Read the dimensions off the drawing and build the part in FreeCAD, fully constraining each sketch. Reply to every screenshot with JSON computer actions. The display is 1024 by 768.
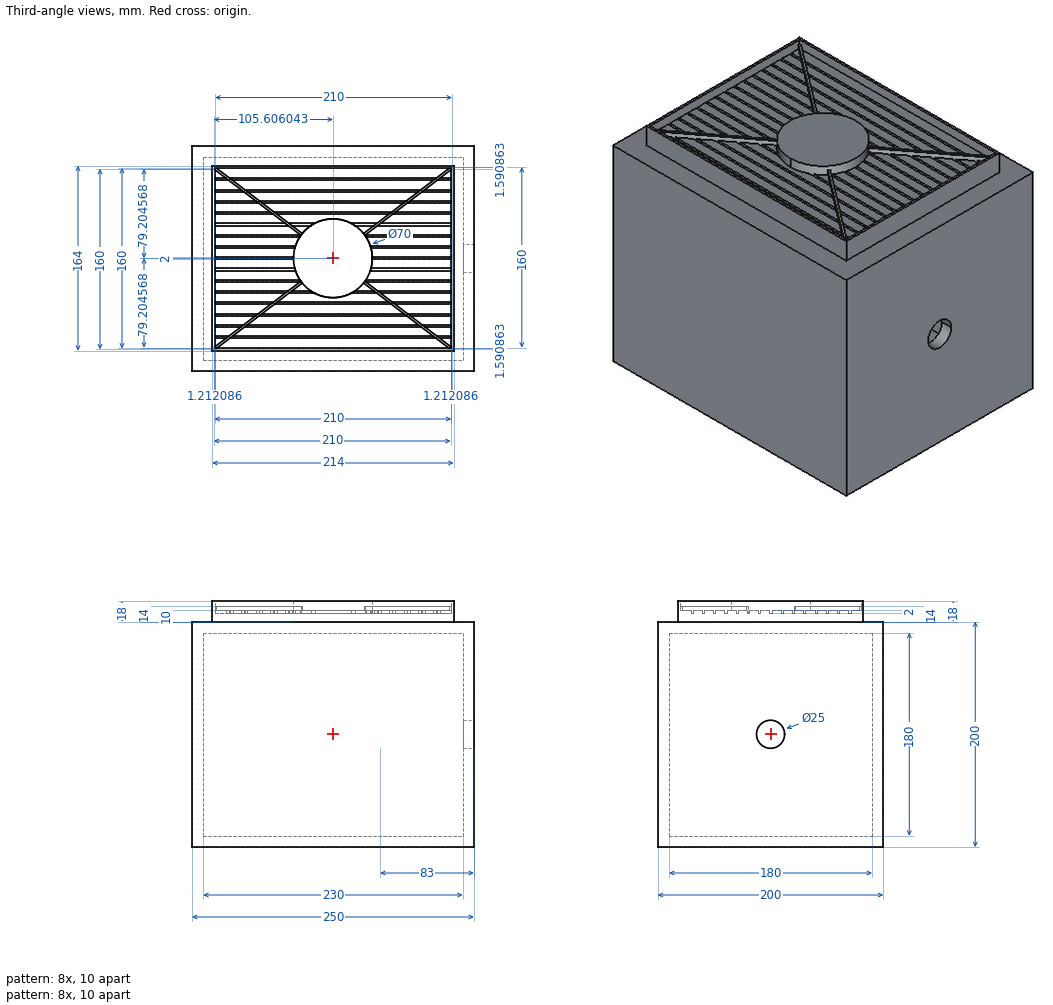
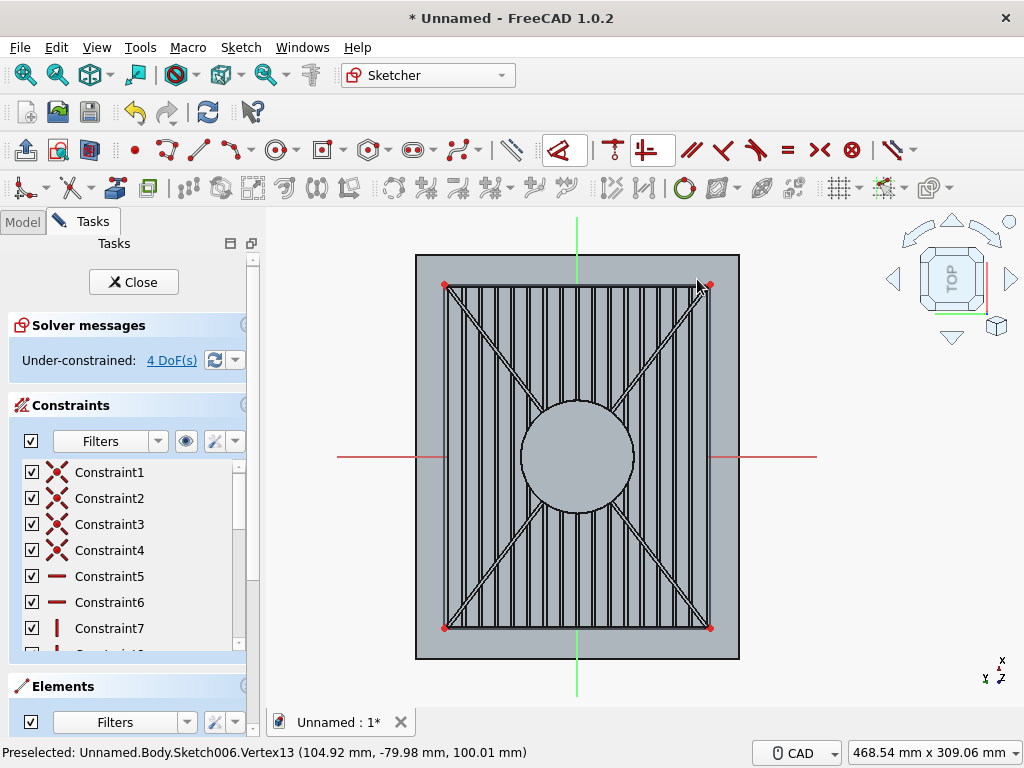
{"action": "scroll", "coordinate": [524, 629], "scroll_direction": "up", "scroll_amount": 10}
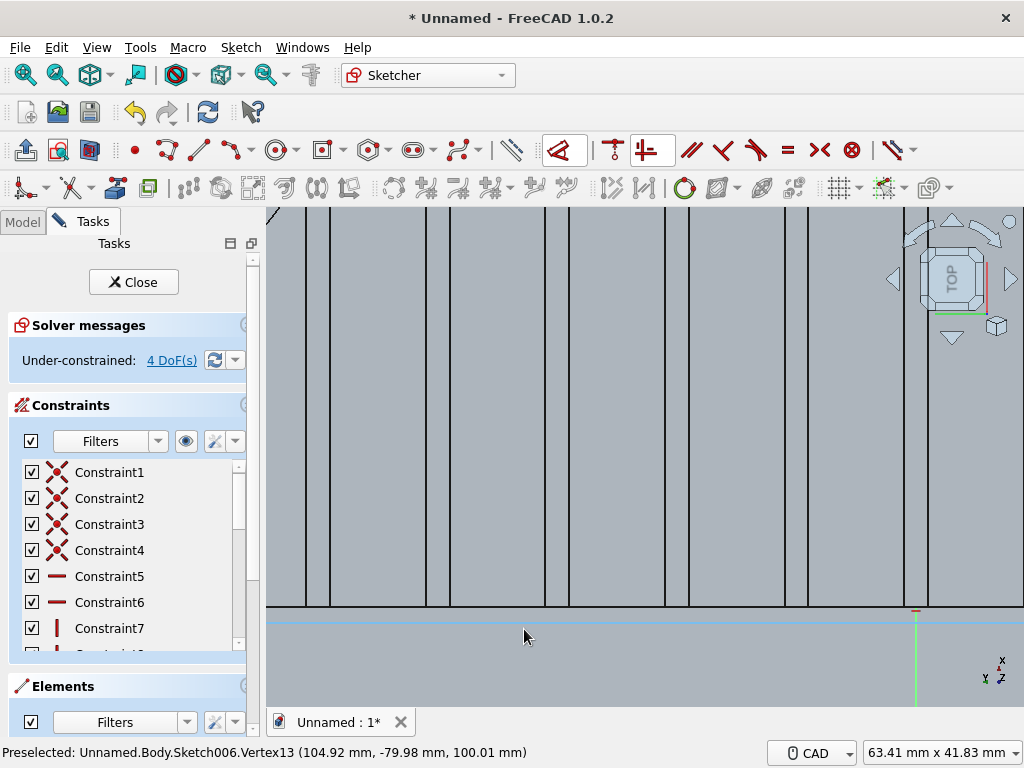
{"action": "left_click", "coordinate": [523, 623]}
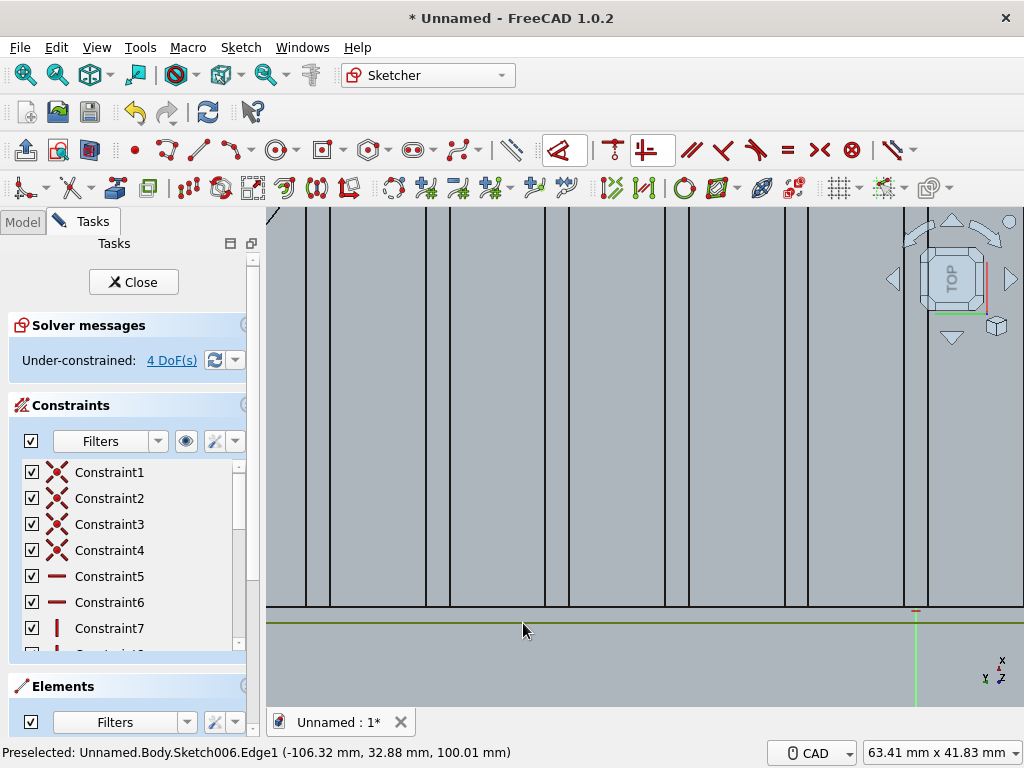
{"action": "left_click", "coordinate": [582, 150]}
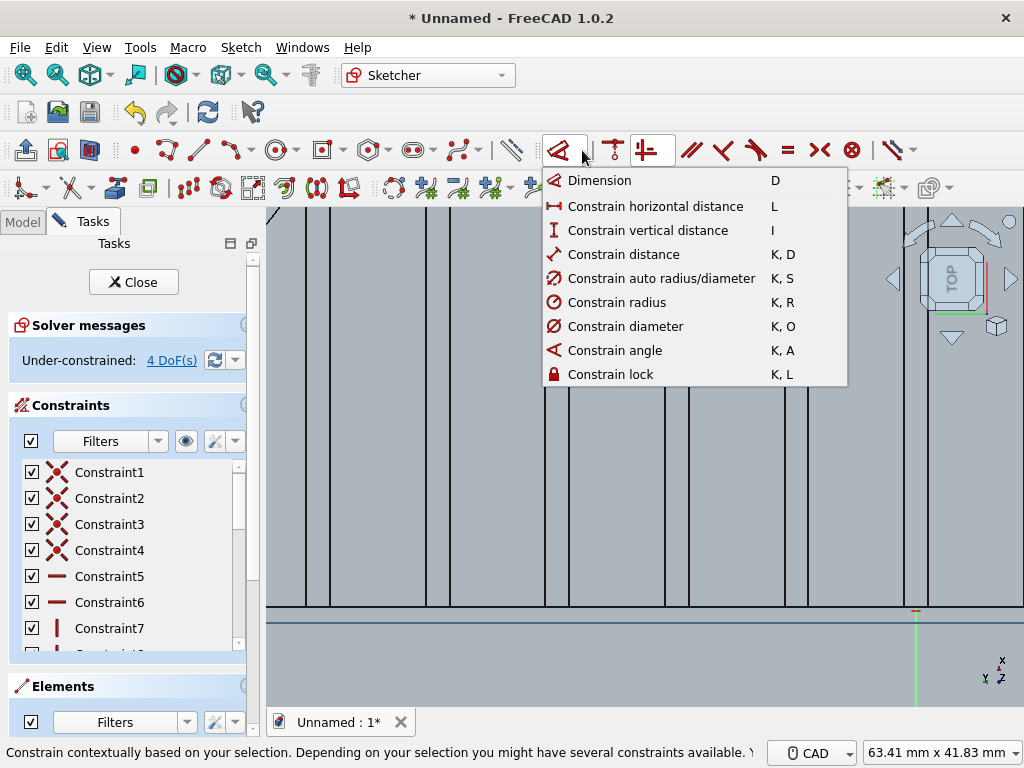
{"action": "left_click", "coordinate": [695, 206]}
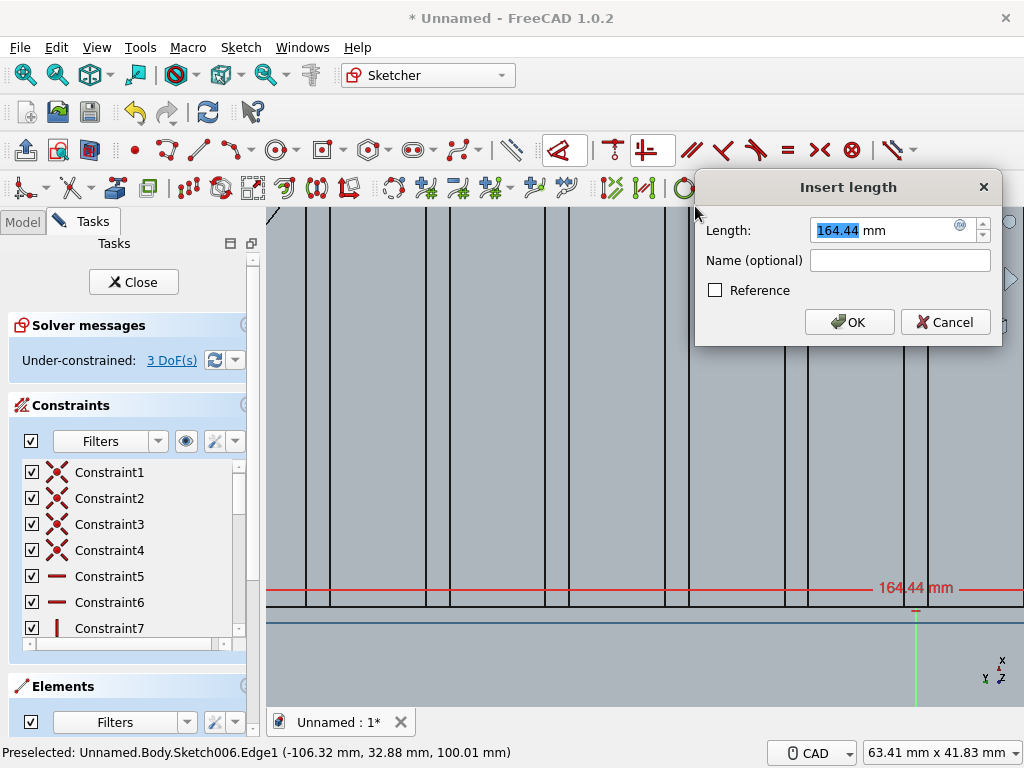
{"action": "type", "text": "164"}
{"action": "key", "text": "Return"}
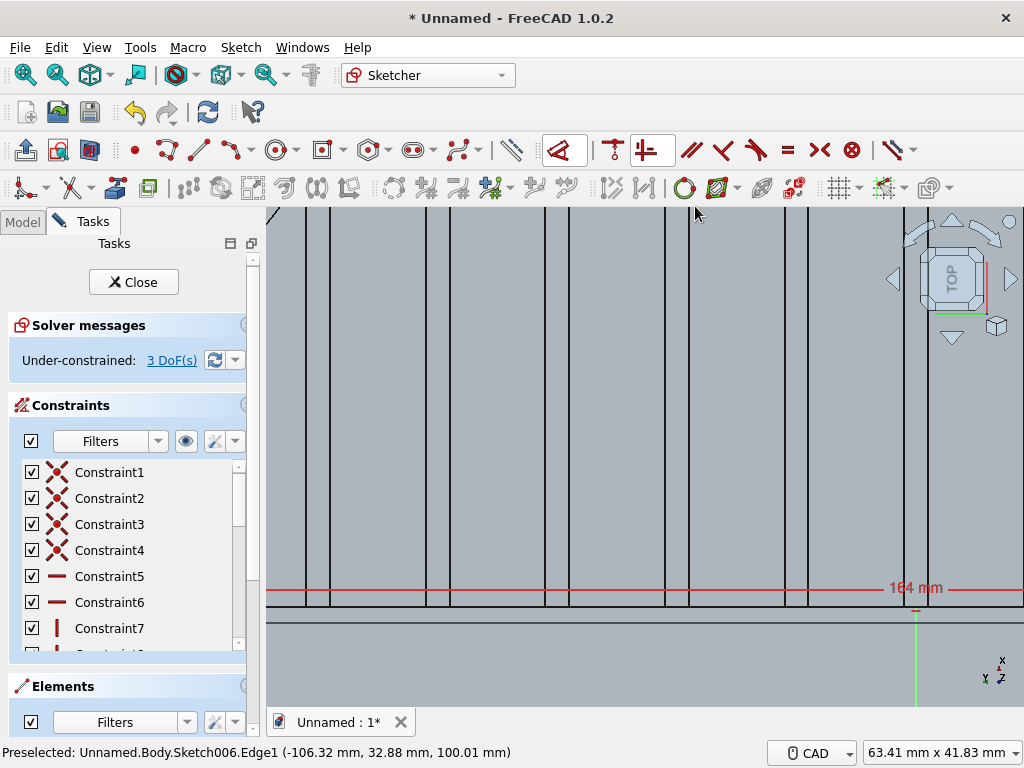
{"action": "scroll", "coordinate": [523, 630], "scroll_direction": "down", "scroll_amount": 10}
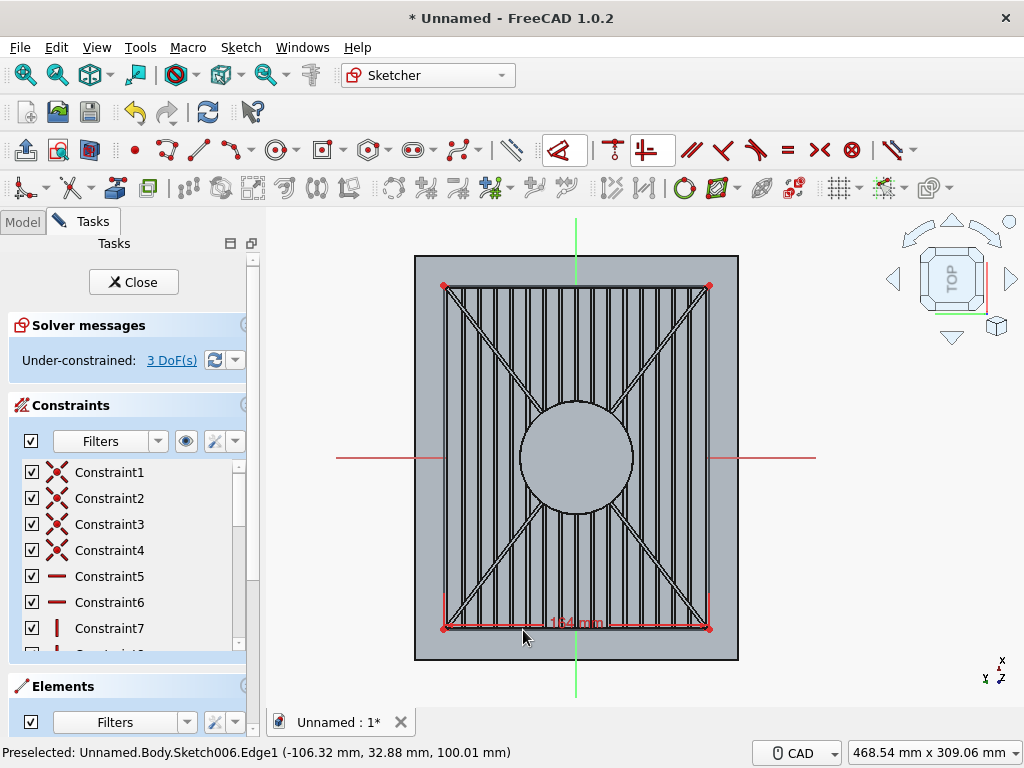
{"action": "scroll", "coordinate": [709, 527], "scroll_direction": "up", "scroll_amount": 8}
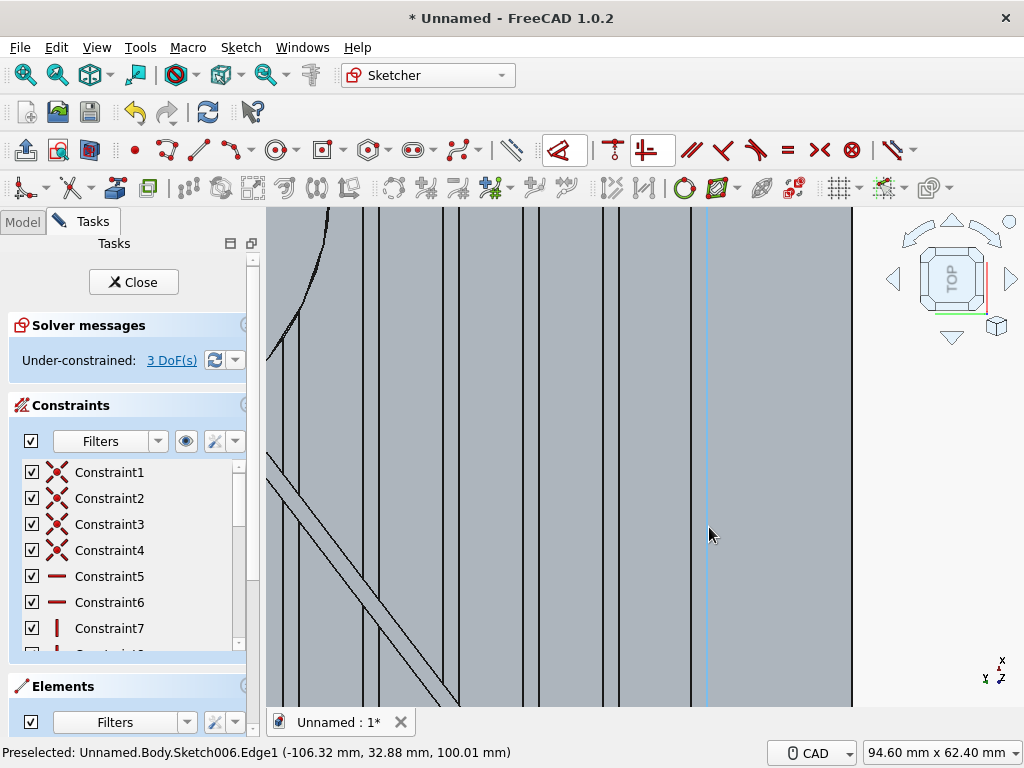
{"action": "left_click", "coordinate": [707, 522]}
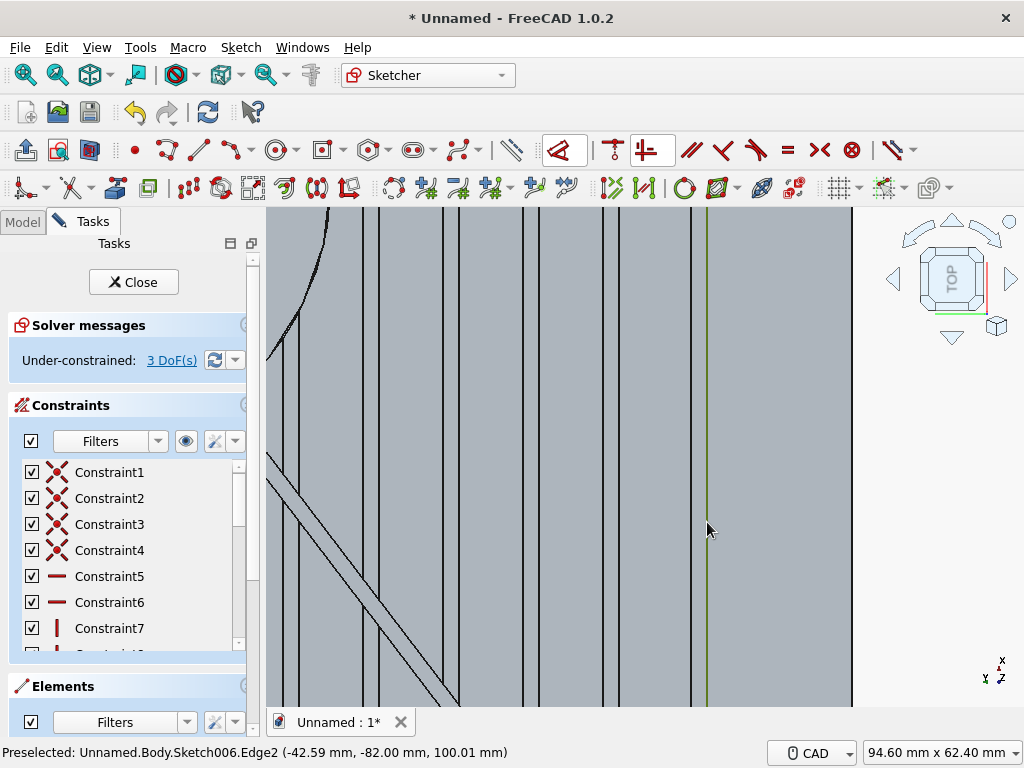
{"action": "key", "text": "i"}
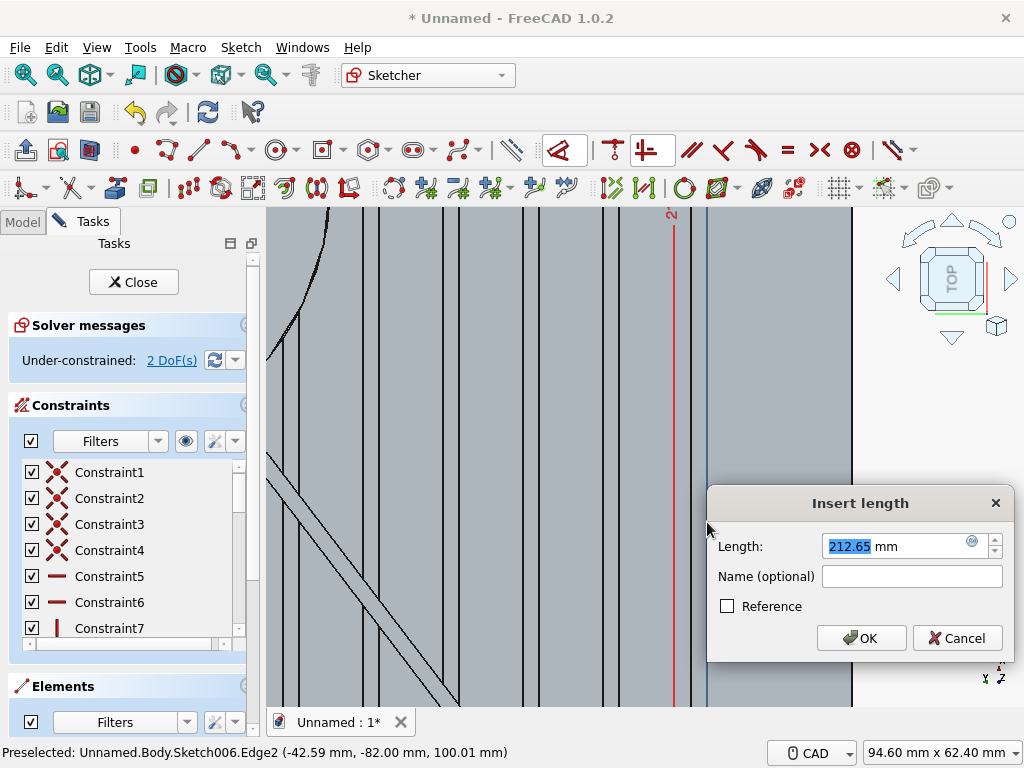
{"action": "type", "text": "214"}
{"action": "key", "text": "Return"}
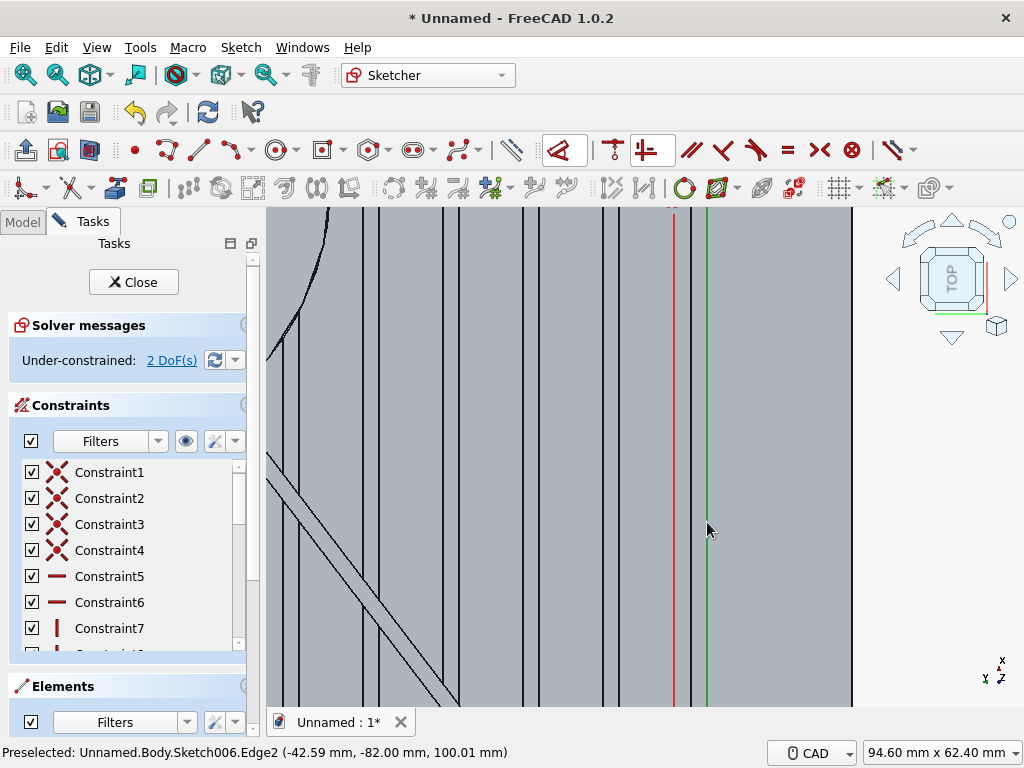
{"action": "scroll", "coordinate": [710, 527], "scroll_direction": "down", "scroll_amount": 8}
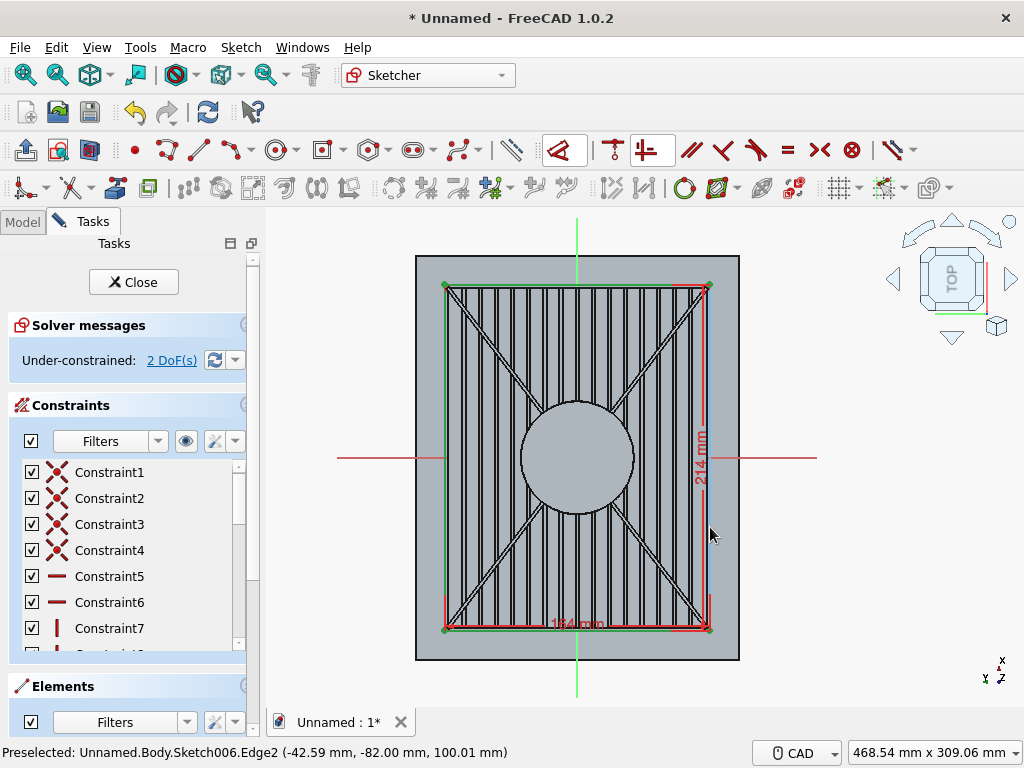
{"action": "scroll", "coordinate": [526, 628], "scroll_direction": "up", "scroll_amount": 8}